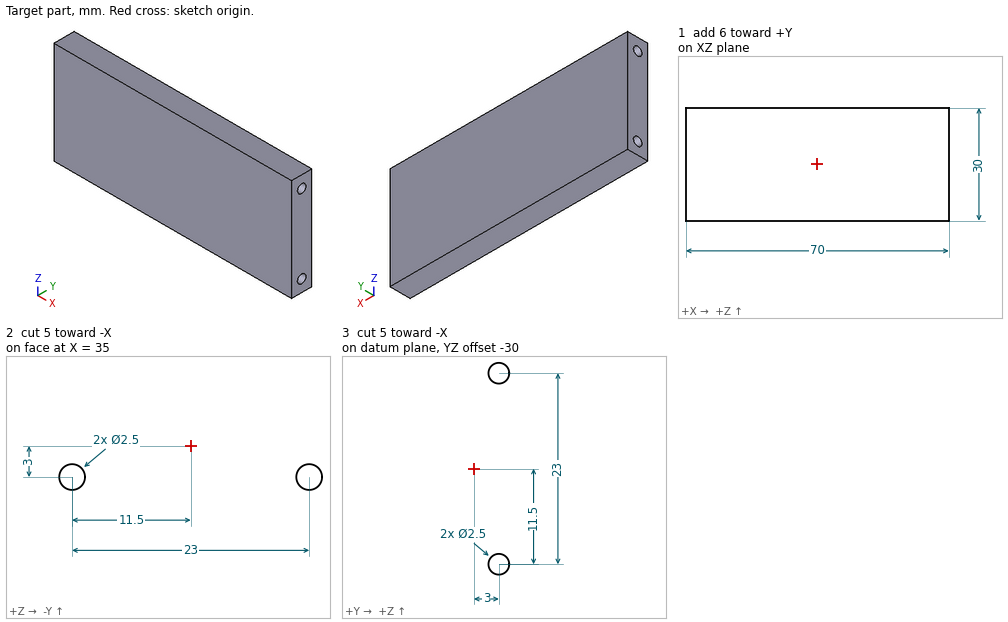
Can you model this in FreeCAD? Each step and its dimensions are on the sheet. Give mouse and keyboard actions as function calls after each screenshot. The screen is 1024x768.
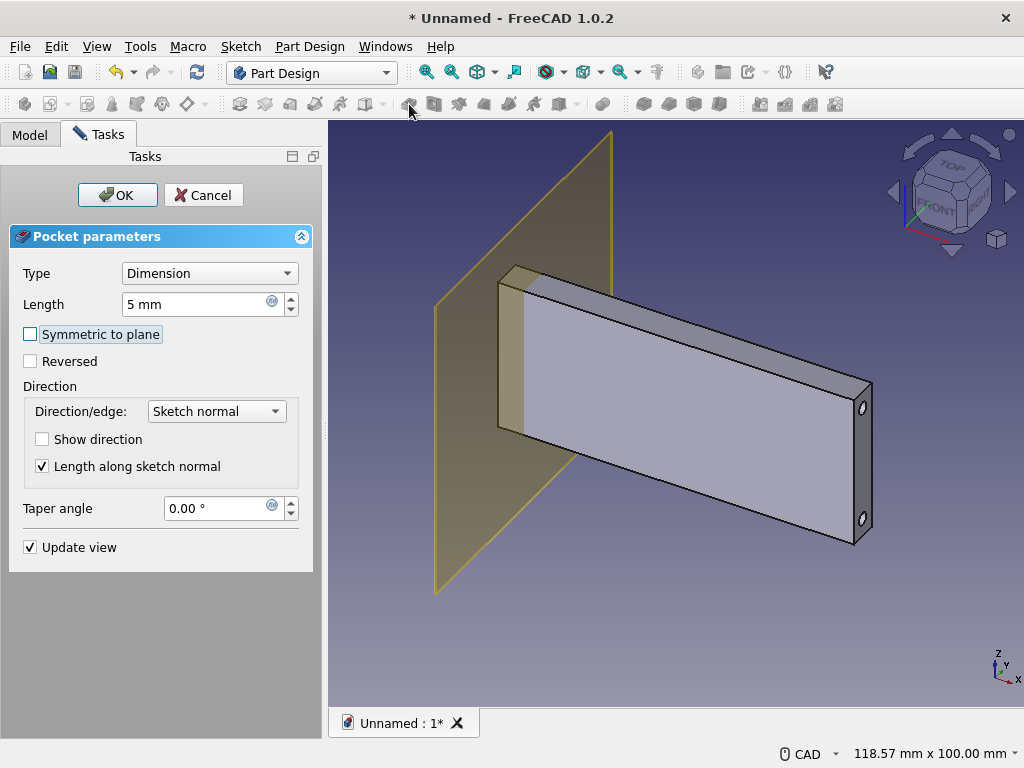
click(118, 195)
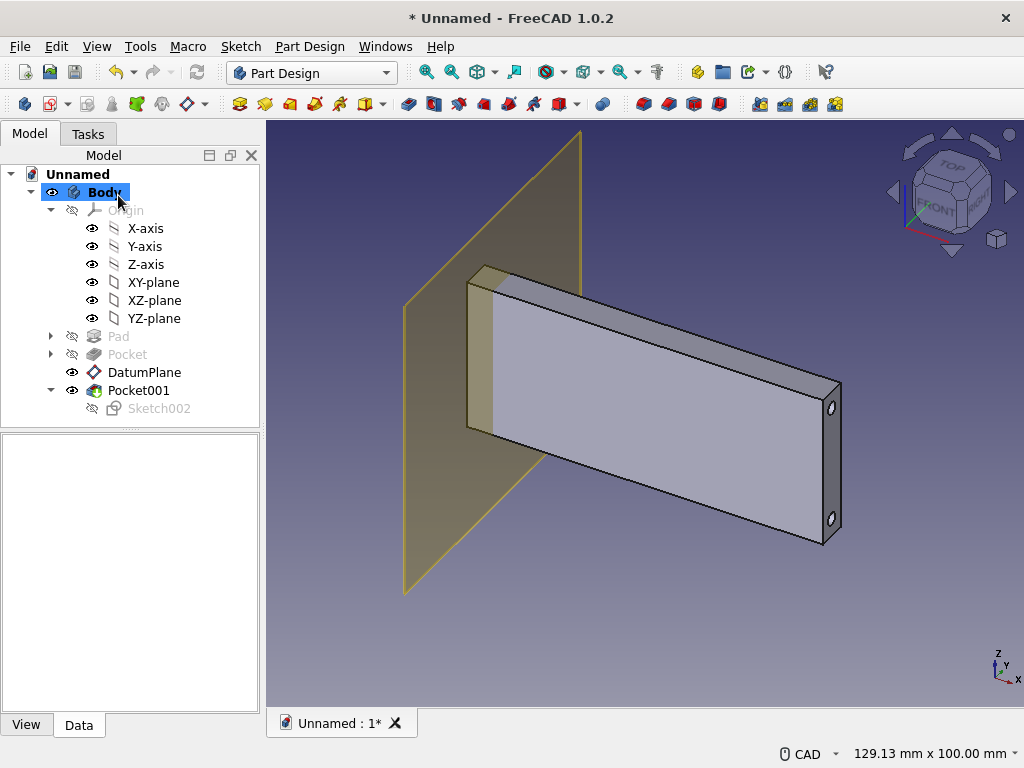
click(117, 372)
key(space)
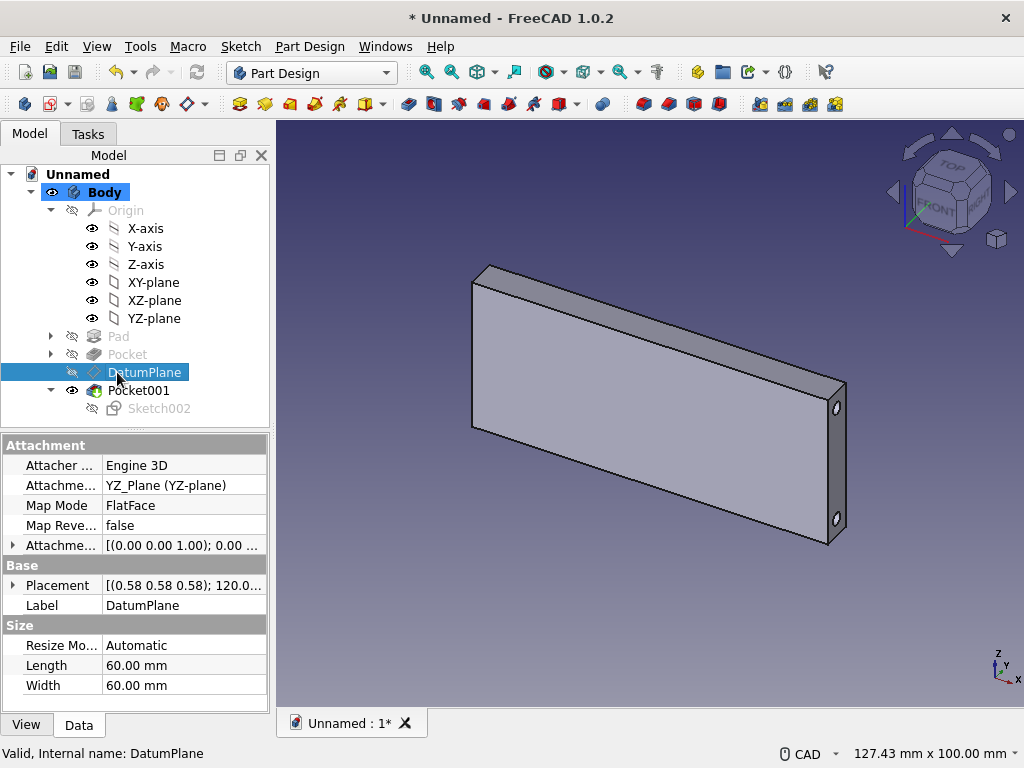
key(0)